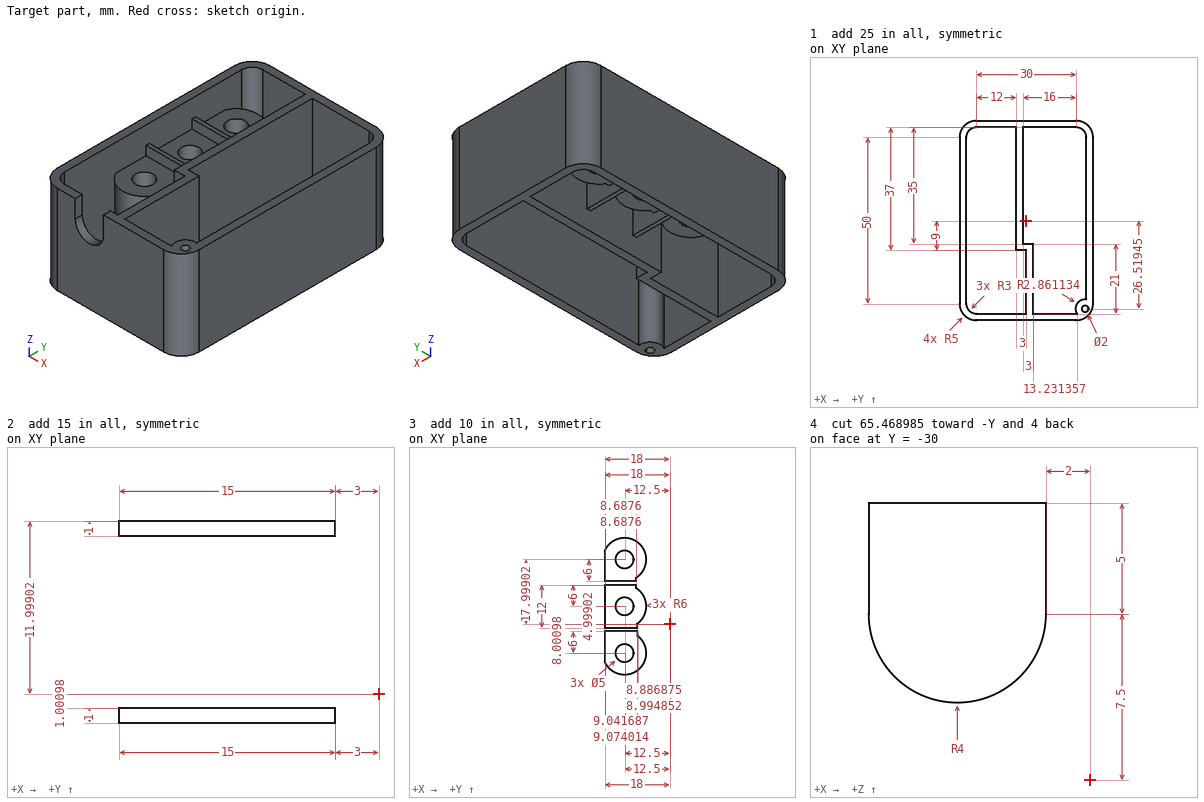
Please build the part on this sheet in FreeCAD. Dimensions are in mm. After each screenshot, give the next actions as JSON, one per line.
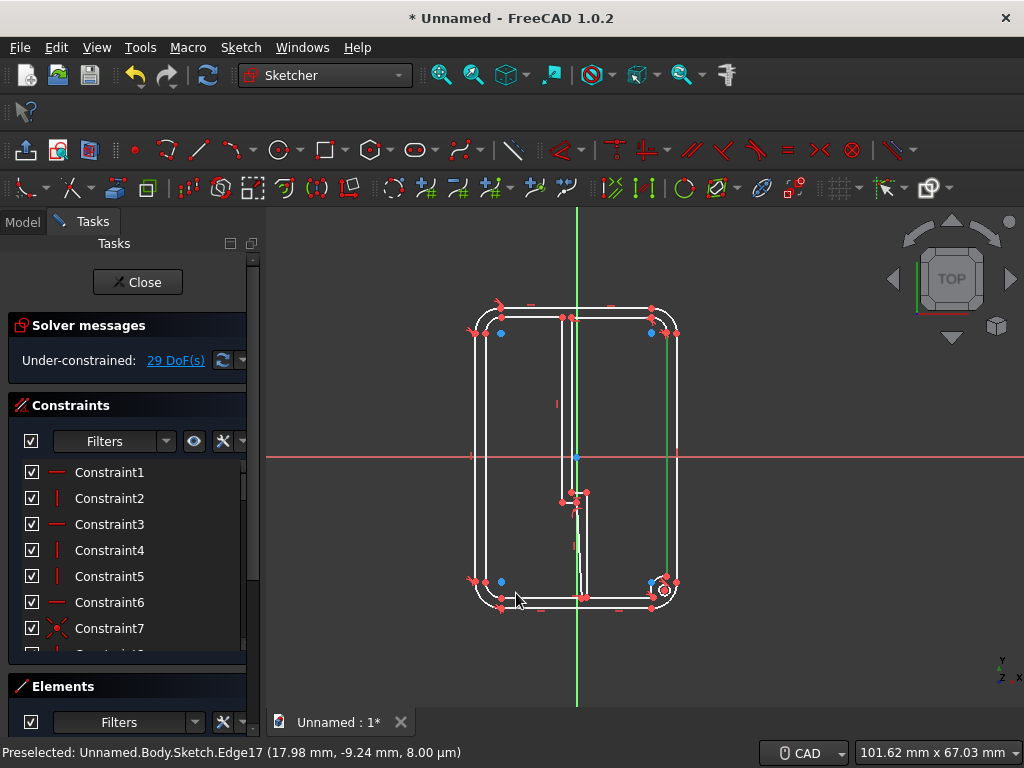
{"action": "scroll", "coordinate": [665, 326], "scroll_direction": "up", "scroll_amount": 4}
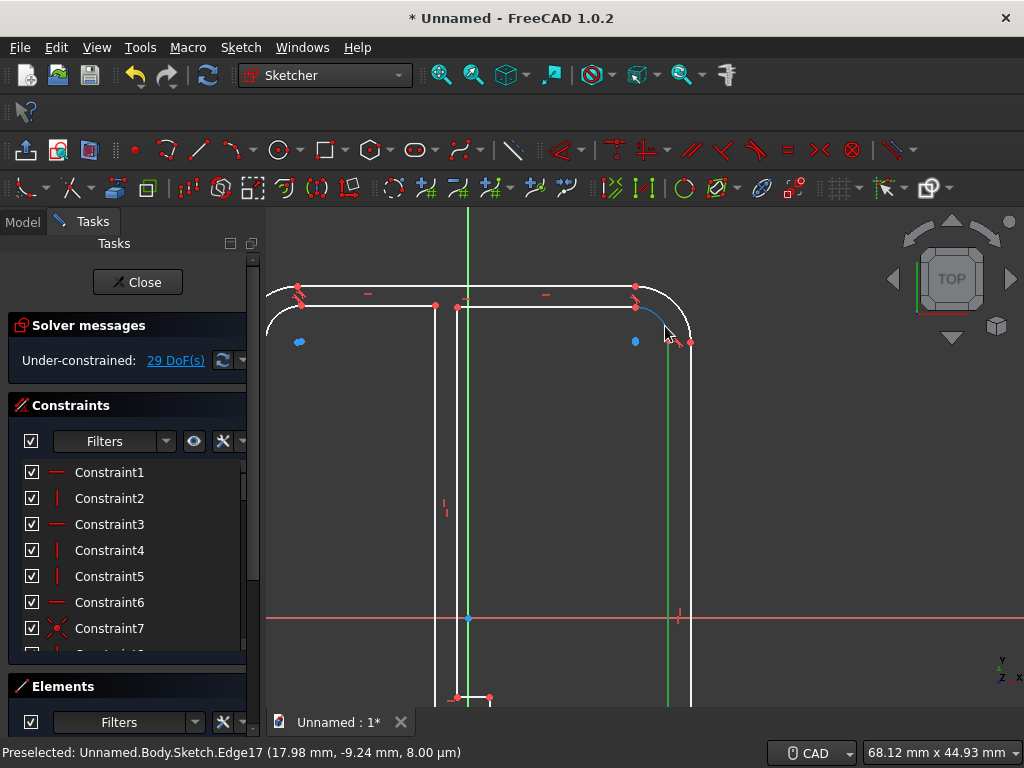
{"action": "left_click", "coordinate": [665, 325]}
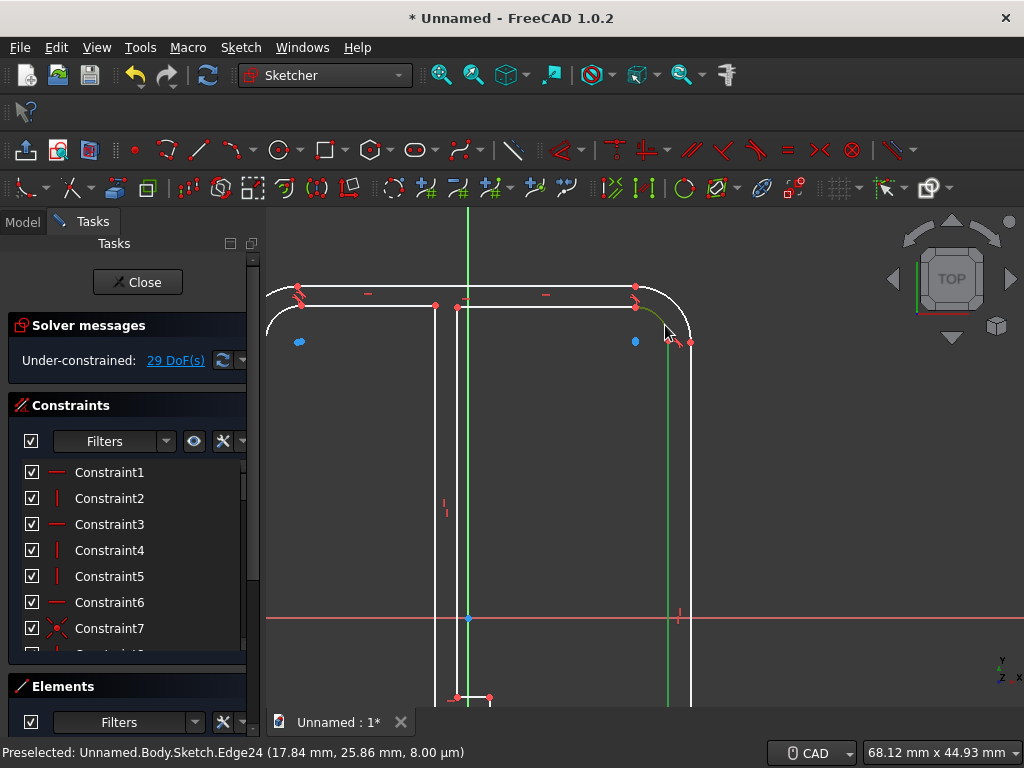
{"action": "left_click", "coordinate": [756, 150]}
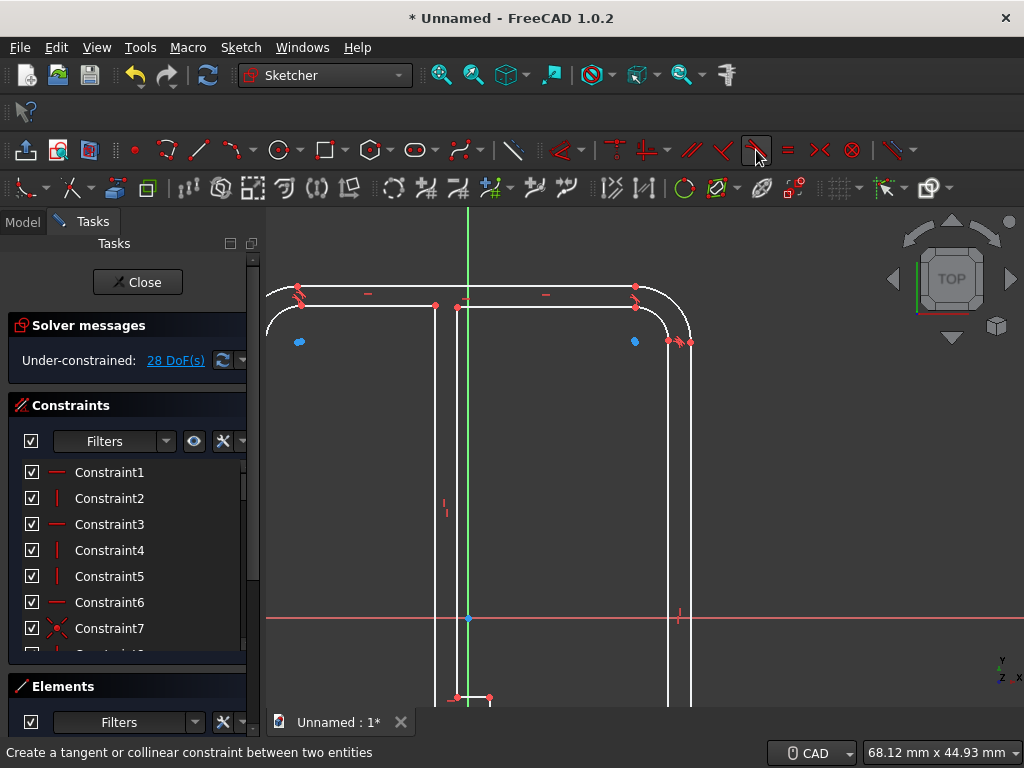
{"action": "left_click", "coordinate": [511, 307]}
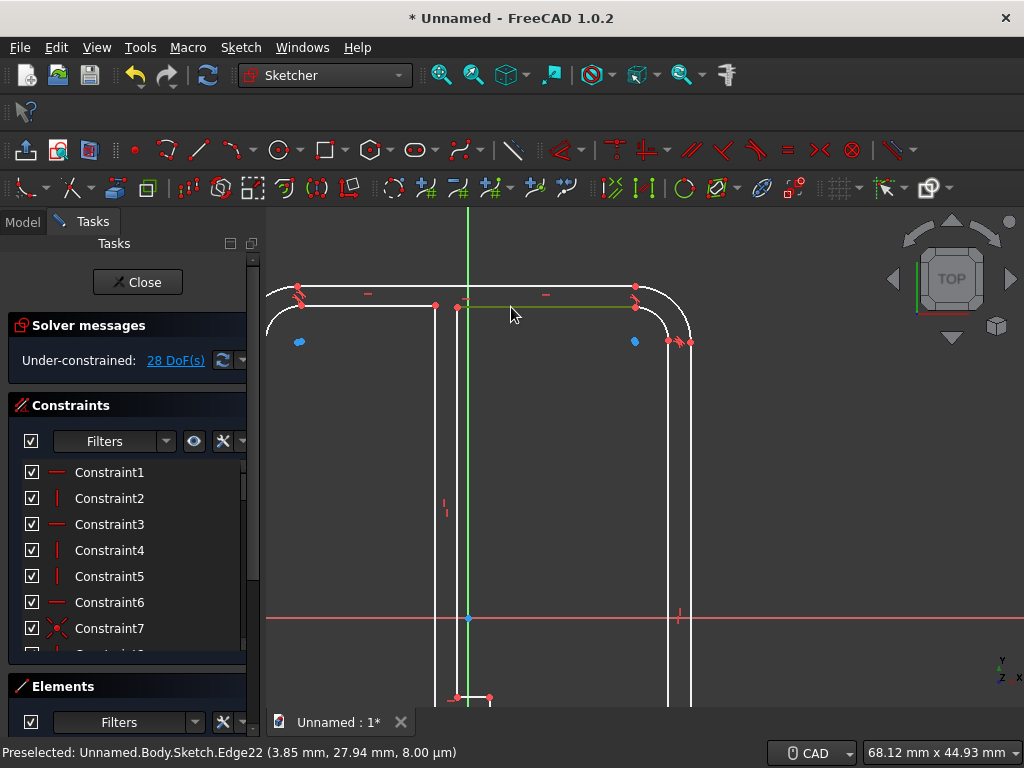
{"action": "left_click", "coordinate": [665, 325]}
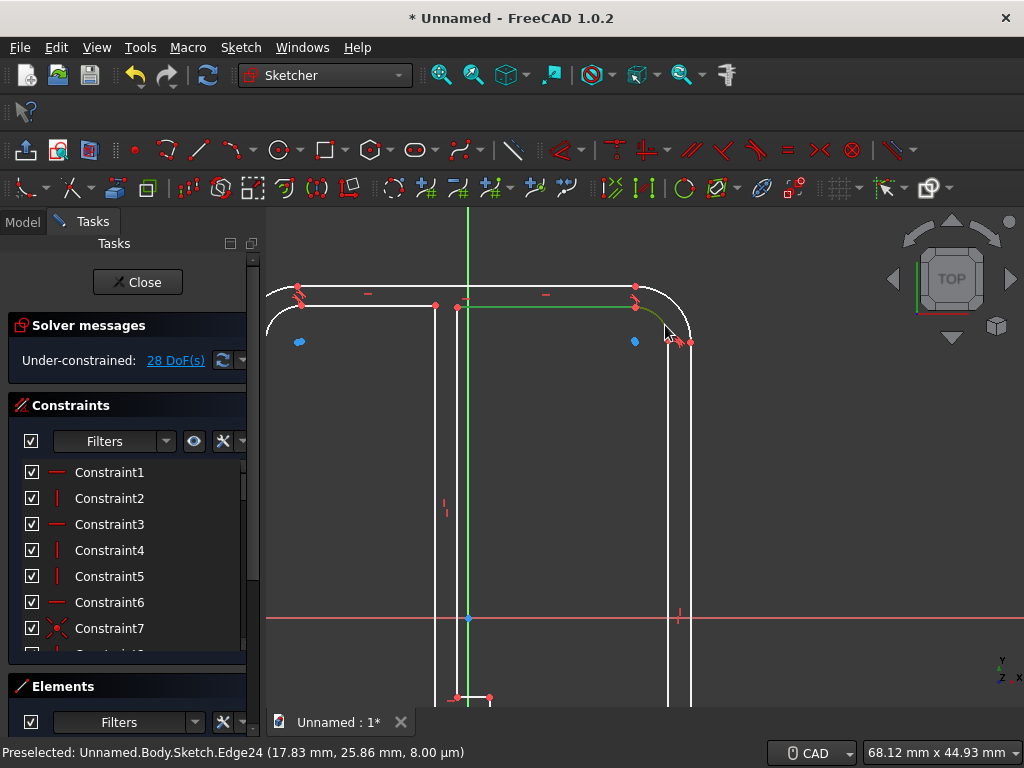
{"action": "left_click", "coordinate": [756, 150]}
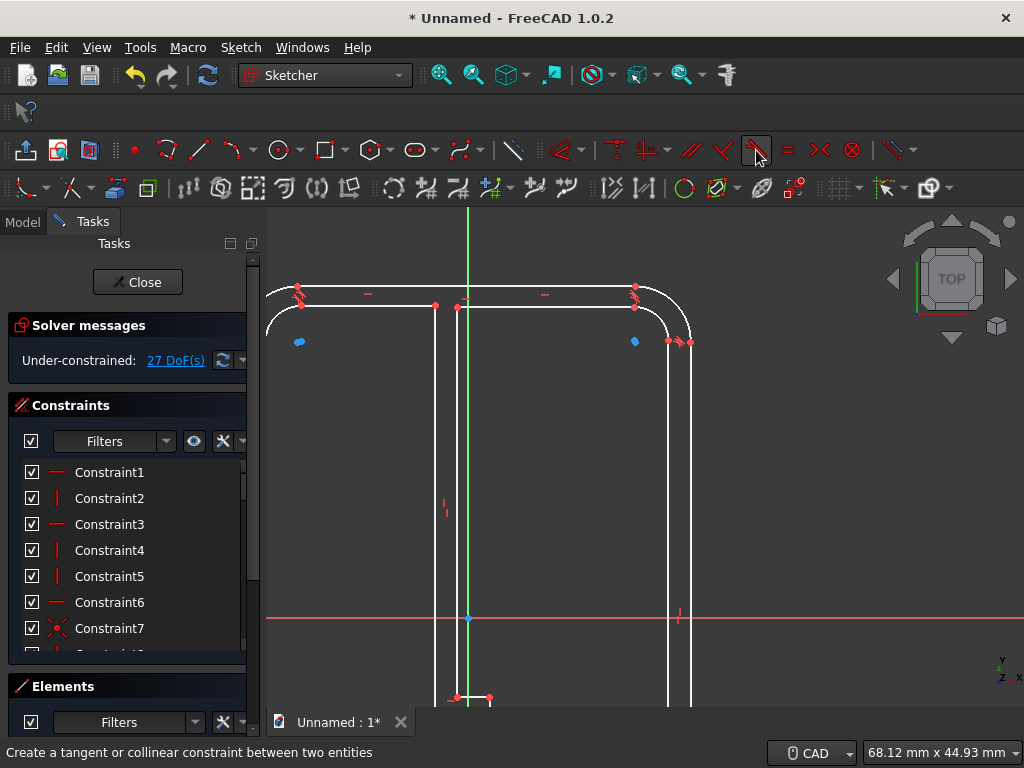
{"action": "scroll", "coordinate": [665, 326], "scroll_direction": "down", "scroll_amount": 4}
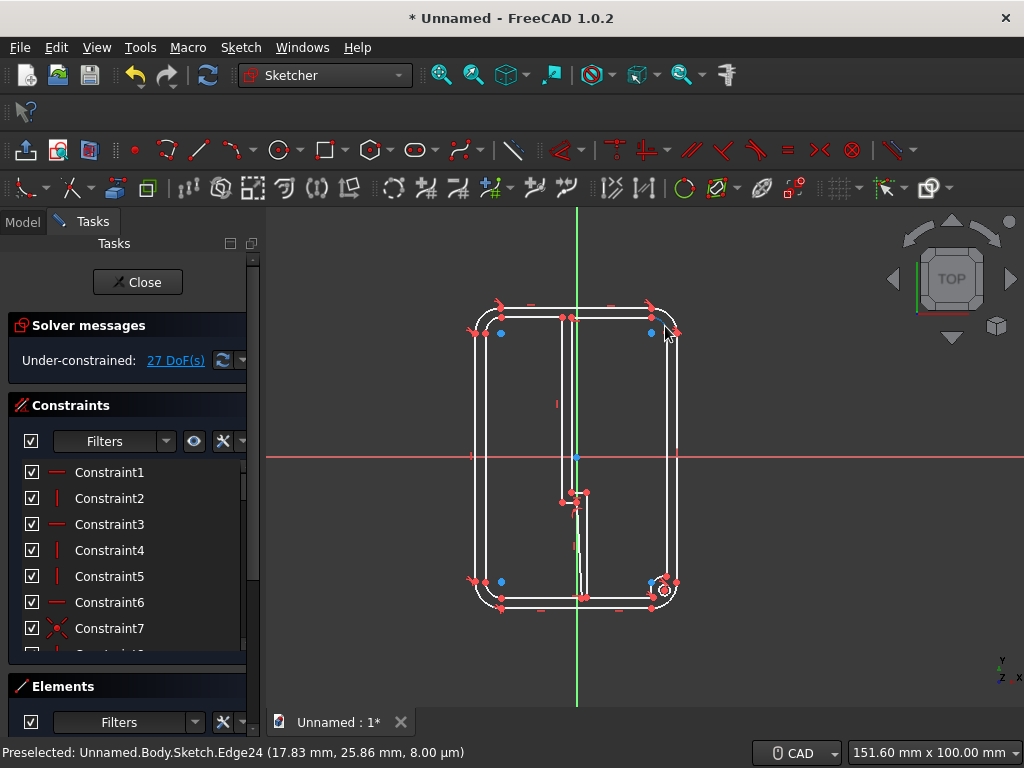
{"action": "scroll", "coordinate": [578, 531], "scroll_direction": "up", "scroll_amount": 3}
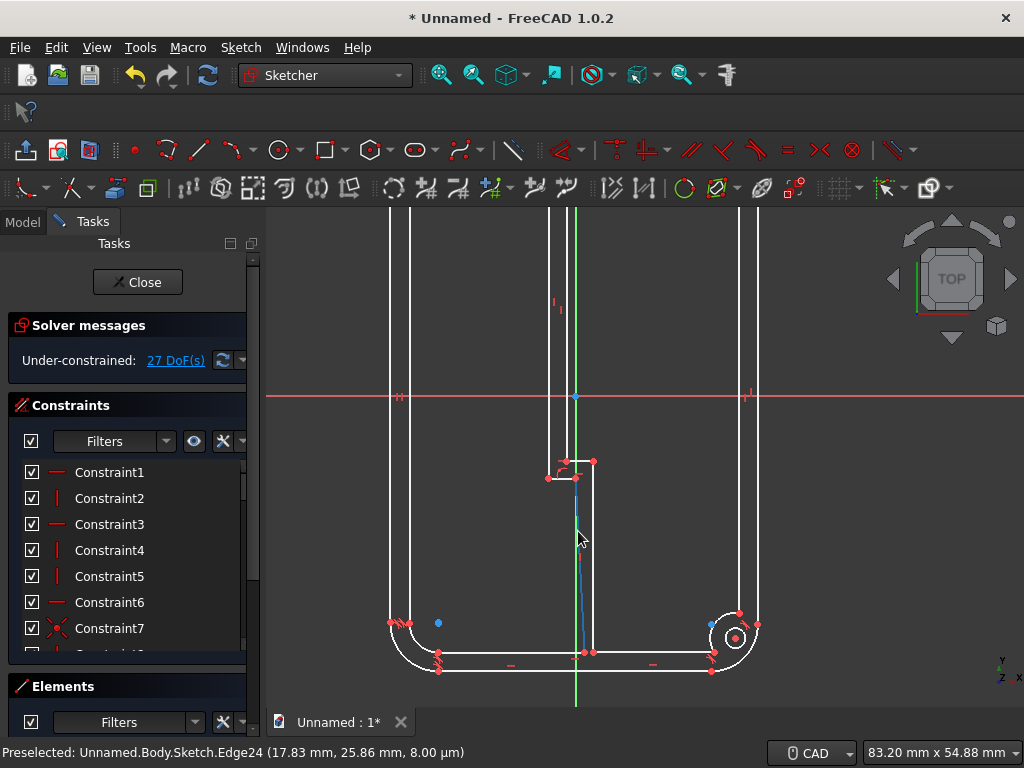
{"action": "left_click", "coordinate": [578, 531]}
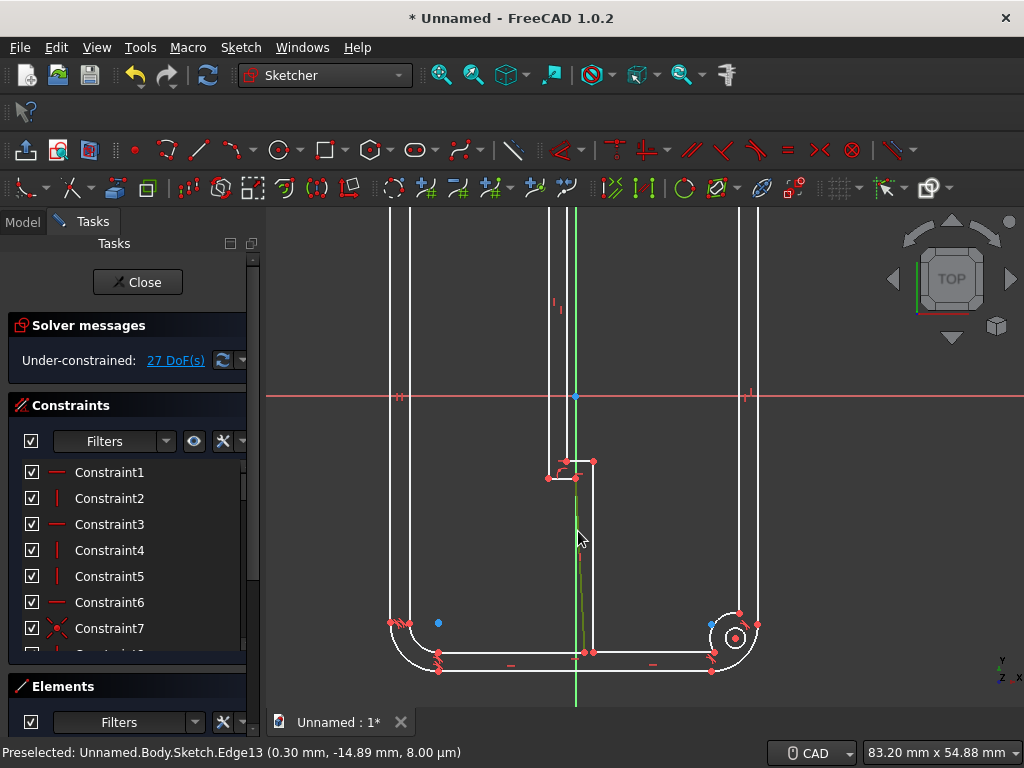
{"action": "left_click", "coordinate": [670, 150]}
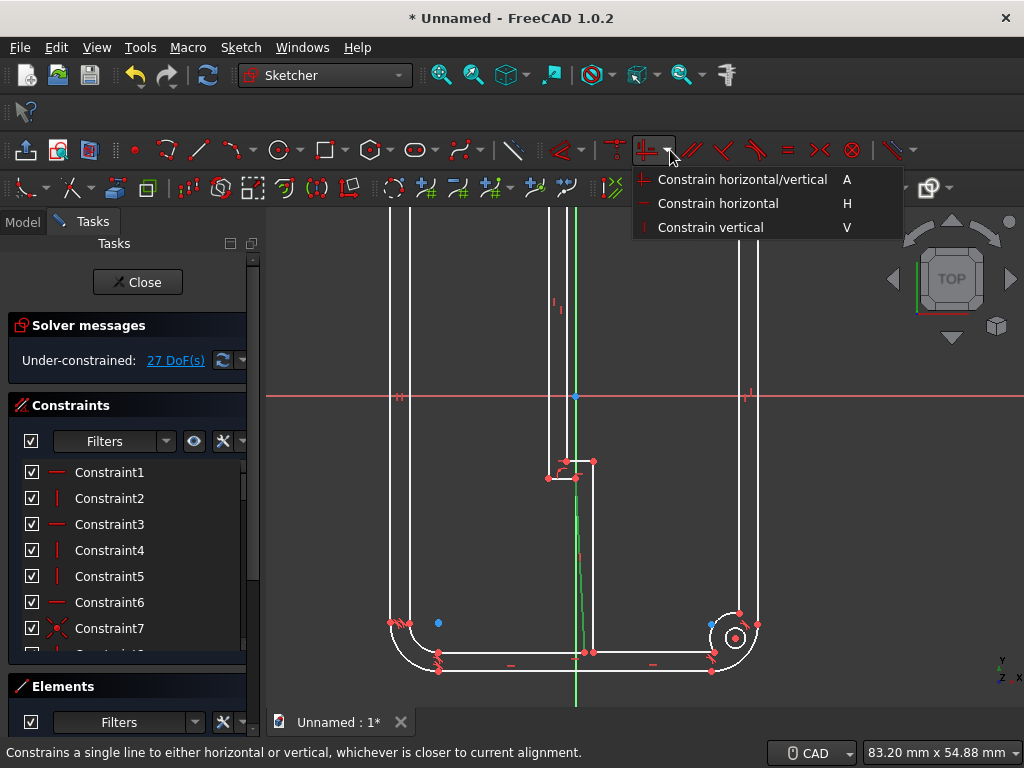
{"action": "left_click", "coordinate": [768, 227]}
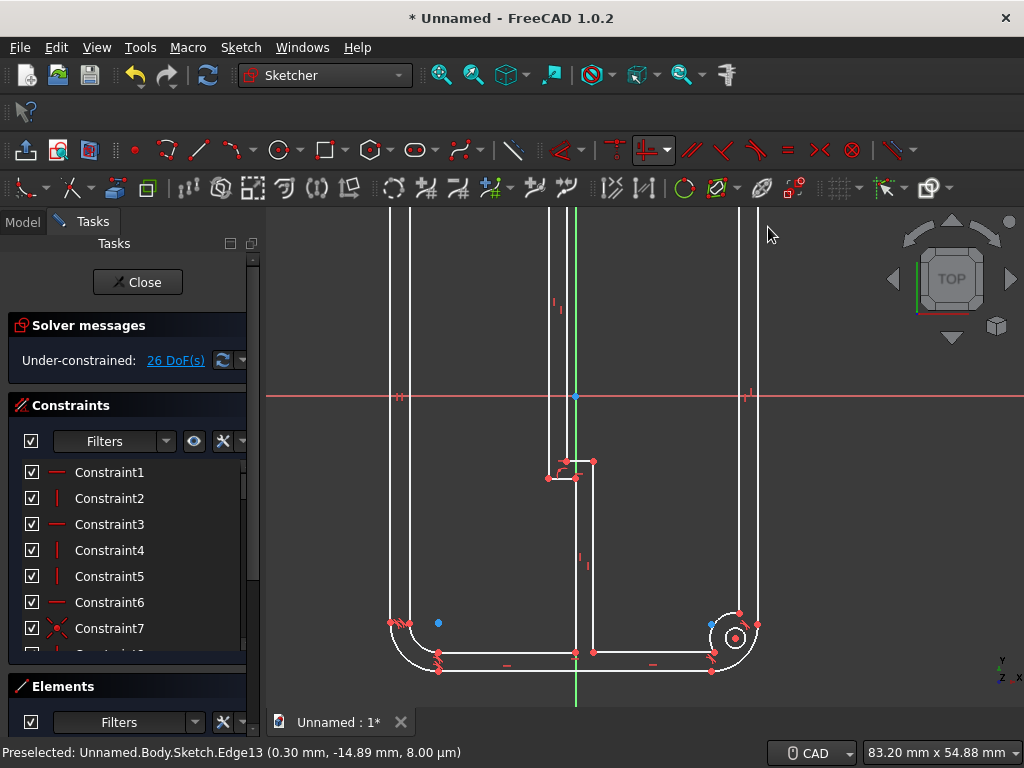
{"action": "scroll", "coordinate": [578, 531], "scroll_direction": "down", "scroll_amount": 3}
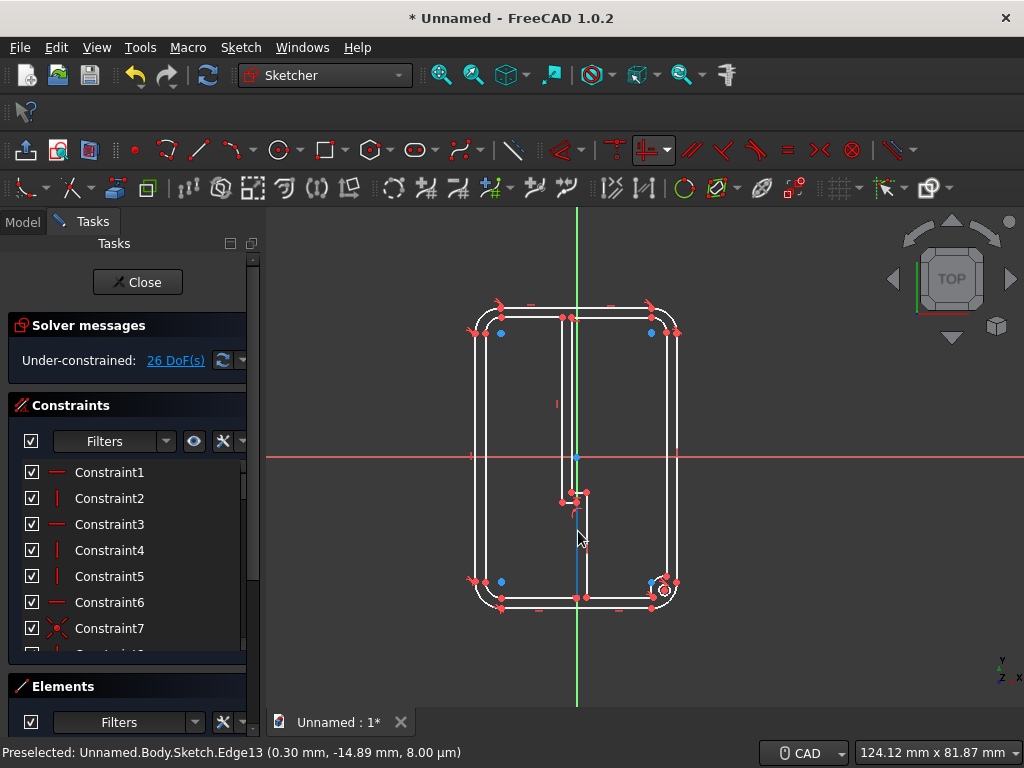
{"action": "scroll", "coordinate": [489, 311], "scroll_direction": "up", "scroll_amount": 2}